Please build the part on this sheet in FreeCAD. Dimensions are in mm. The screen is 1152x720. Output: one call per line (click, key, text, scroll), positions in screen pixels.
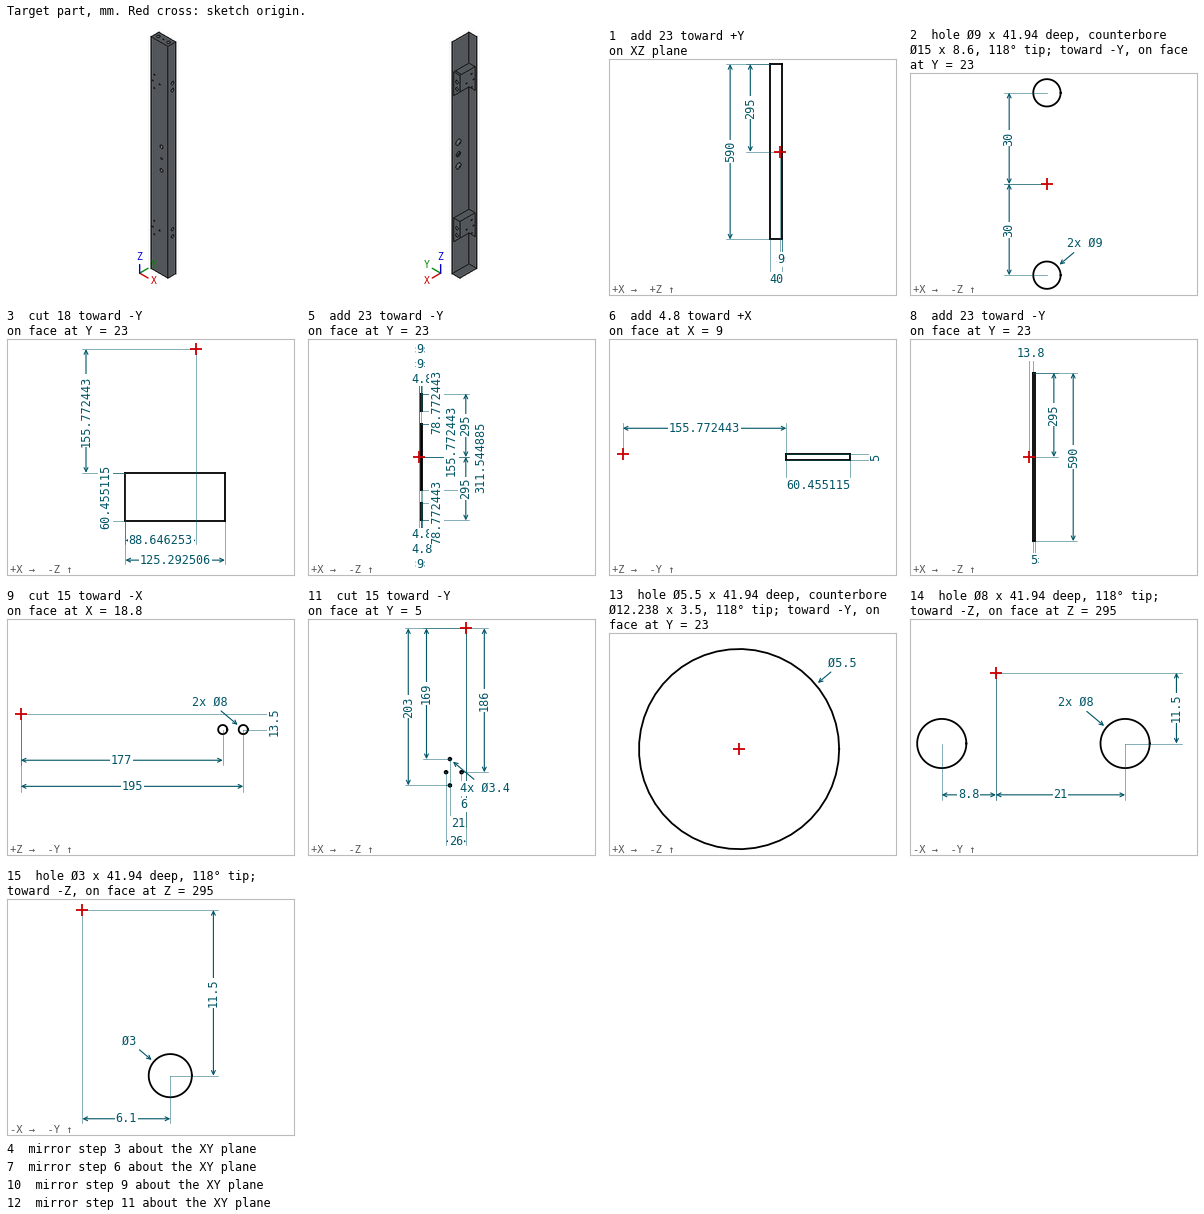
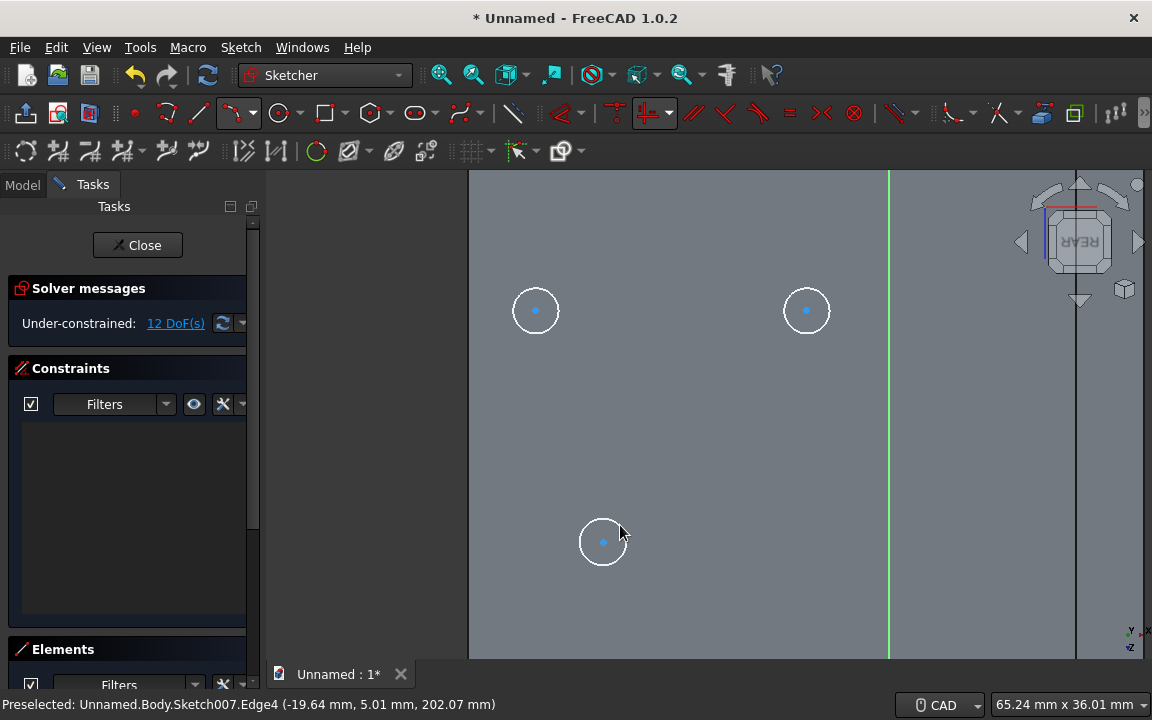
scroll(603, 542, down, 3)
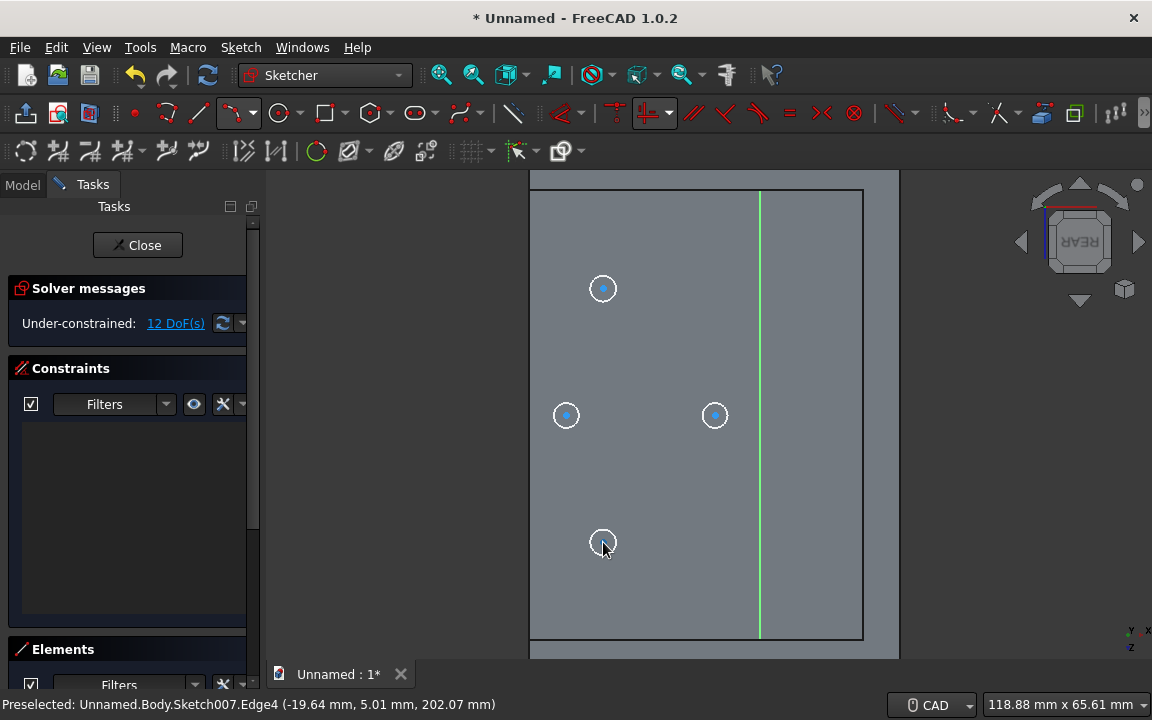
click(612, 280)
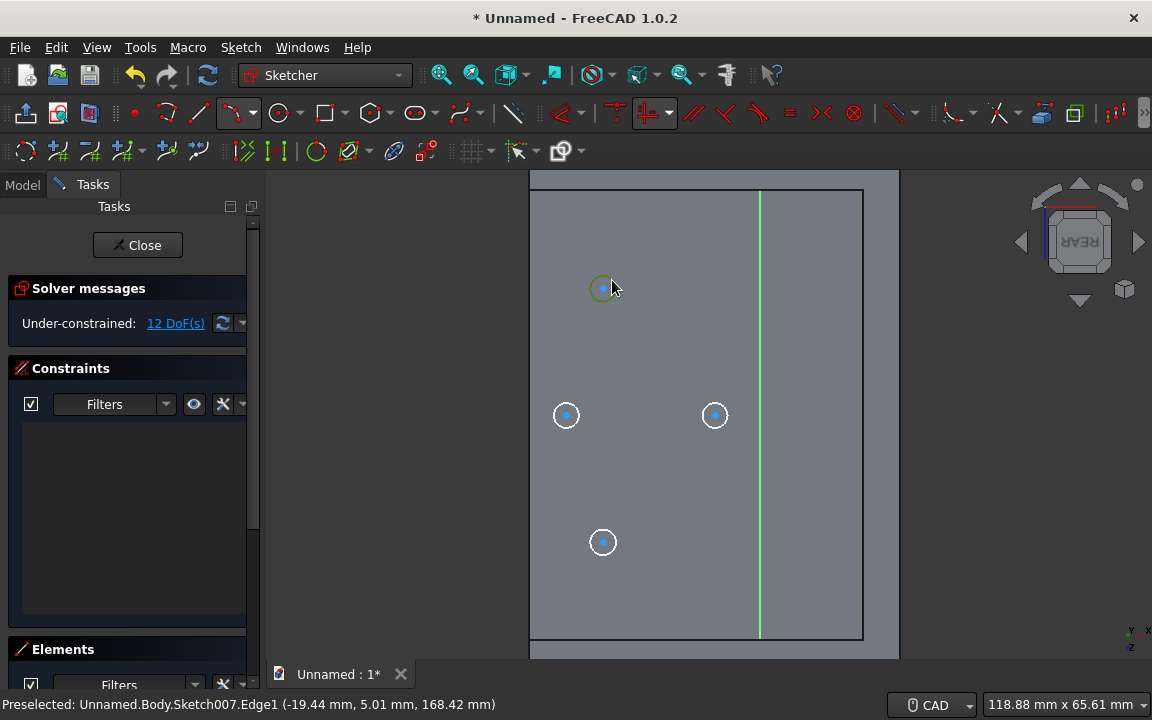
click(724, 407)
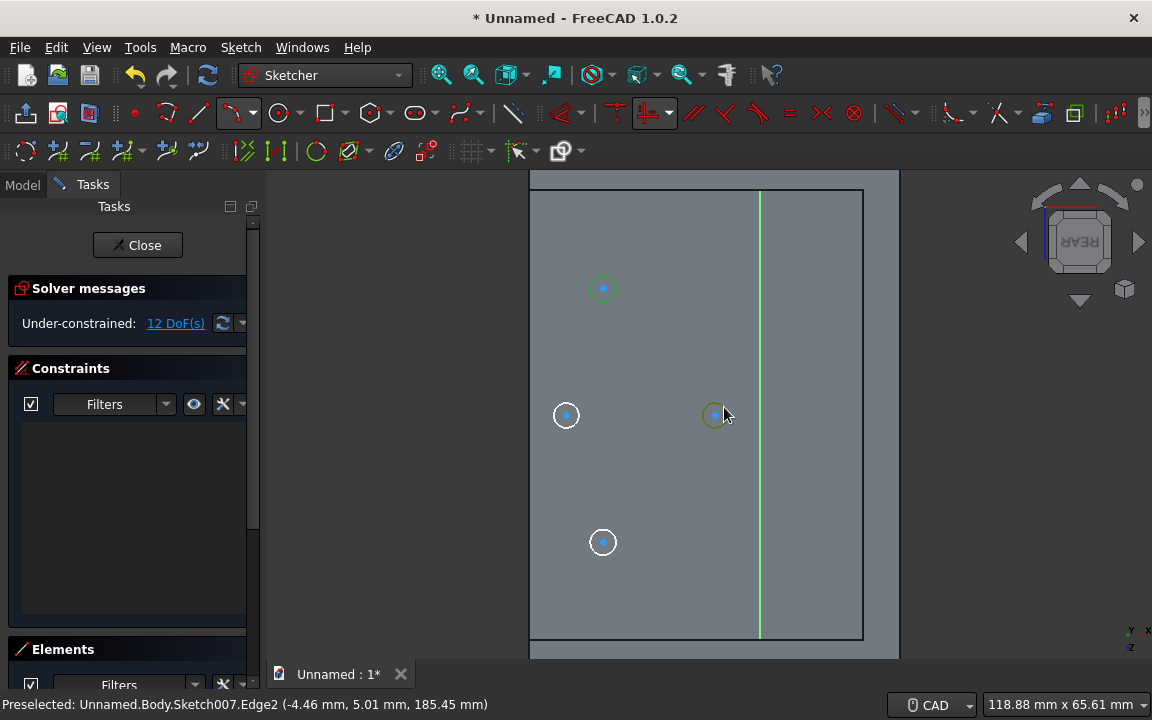
click(575, 407)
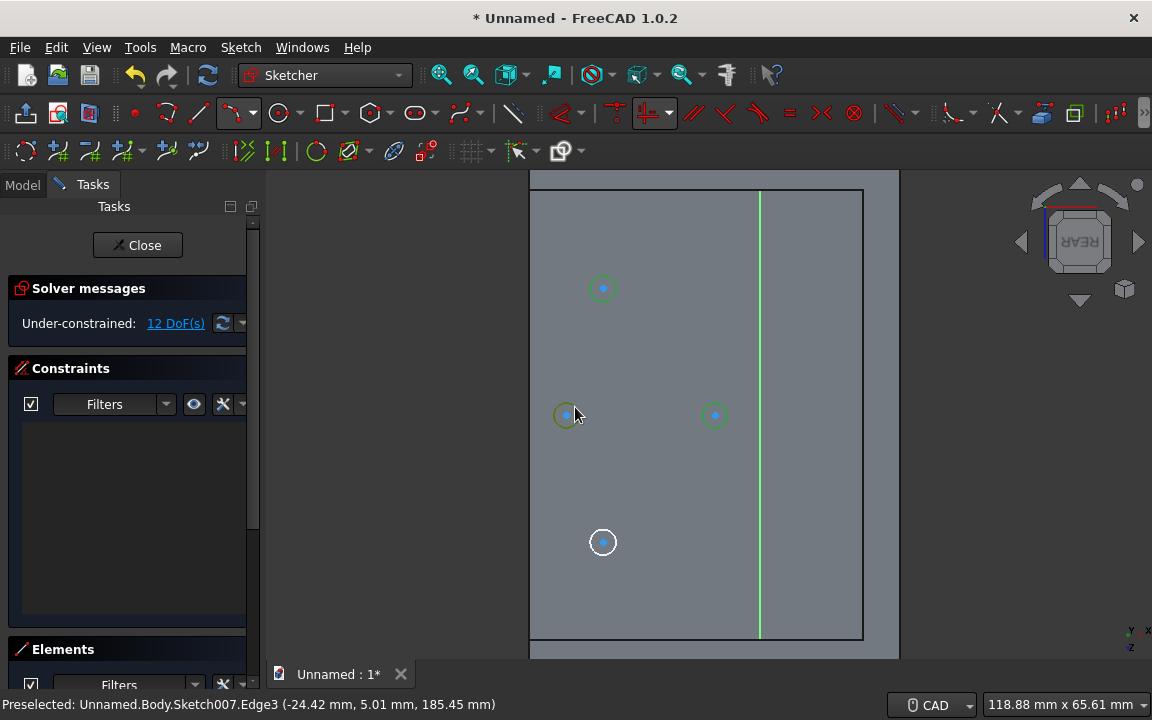
click(612, 533)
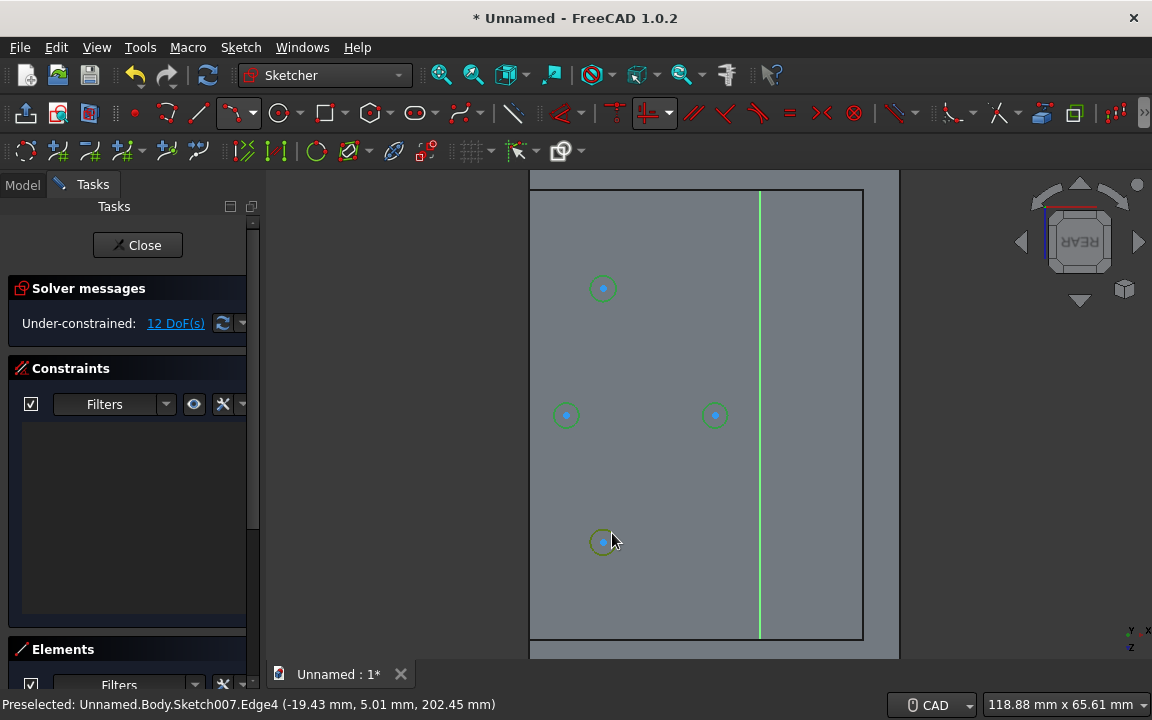
click(790, 114)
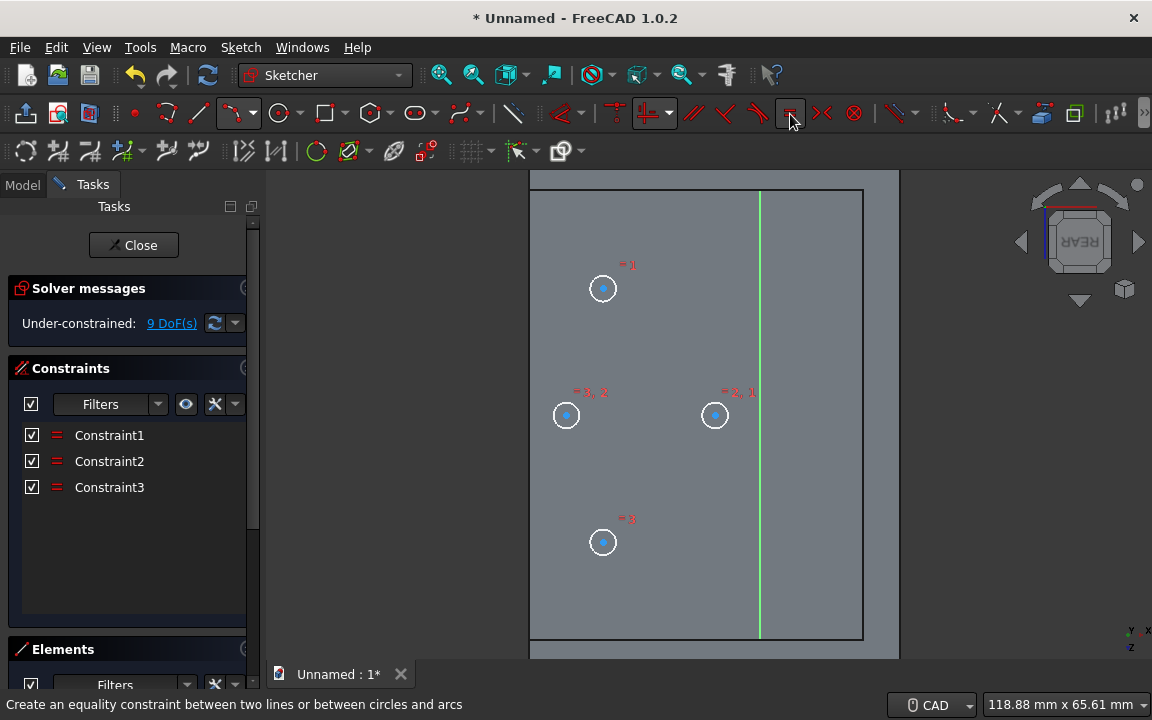
click(715, 415)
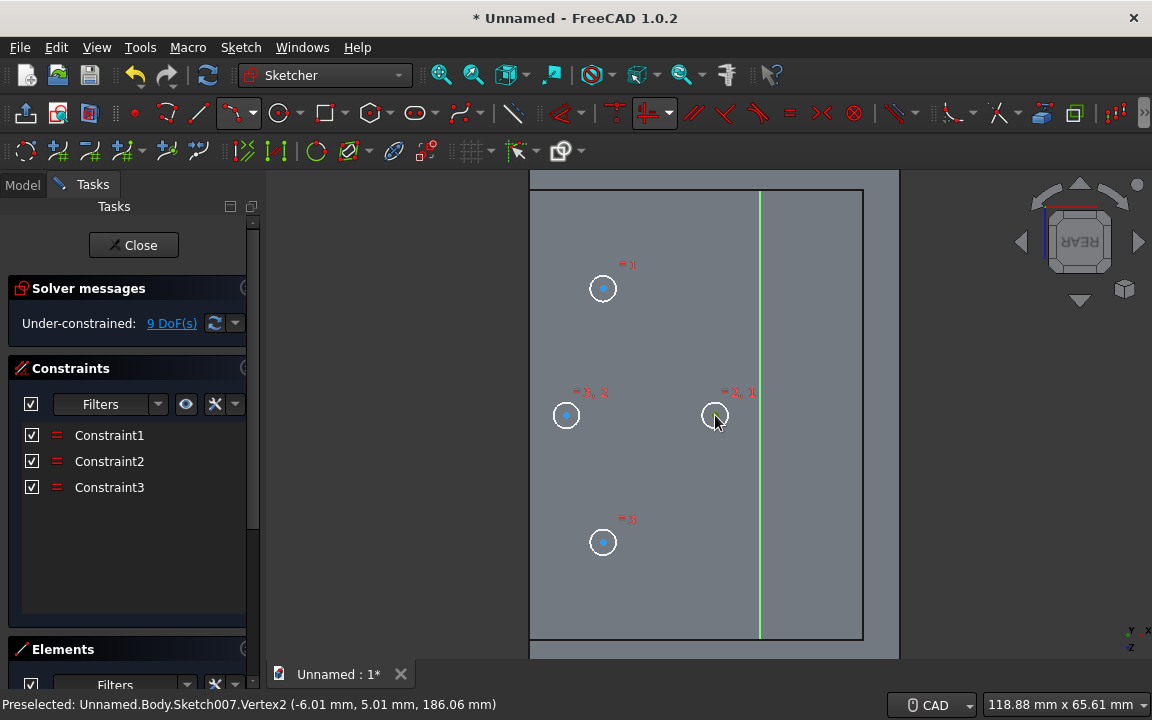
click(566, 415)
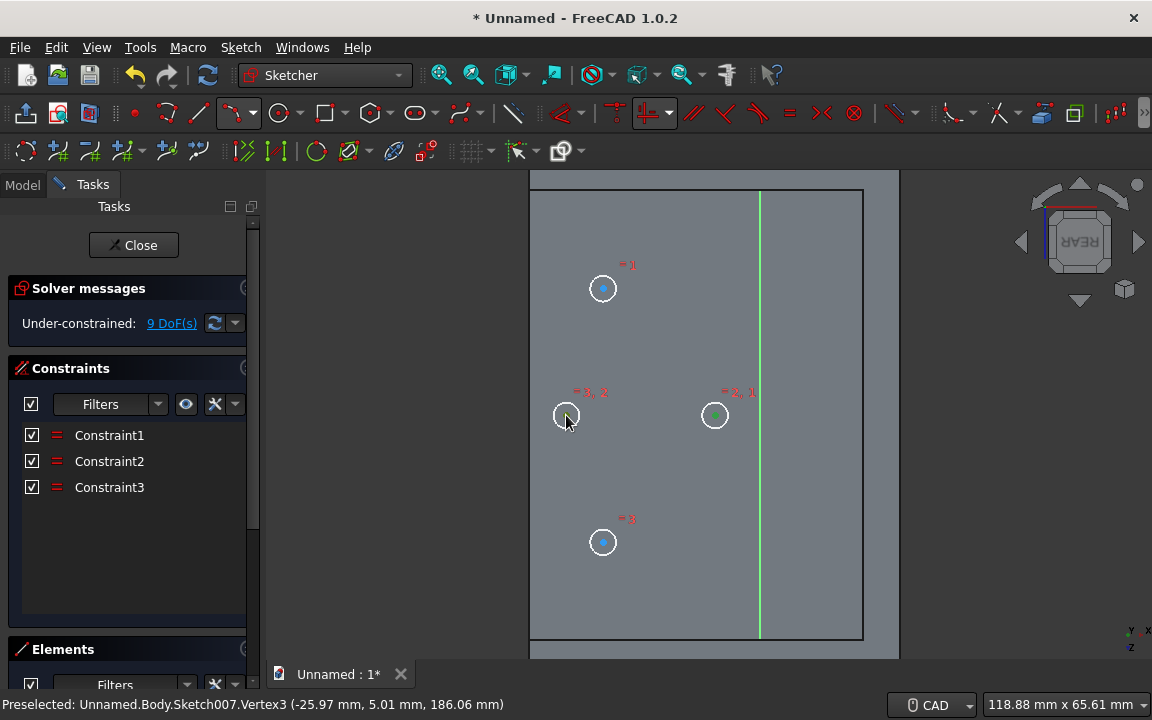
key(h)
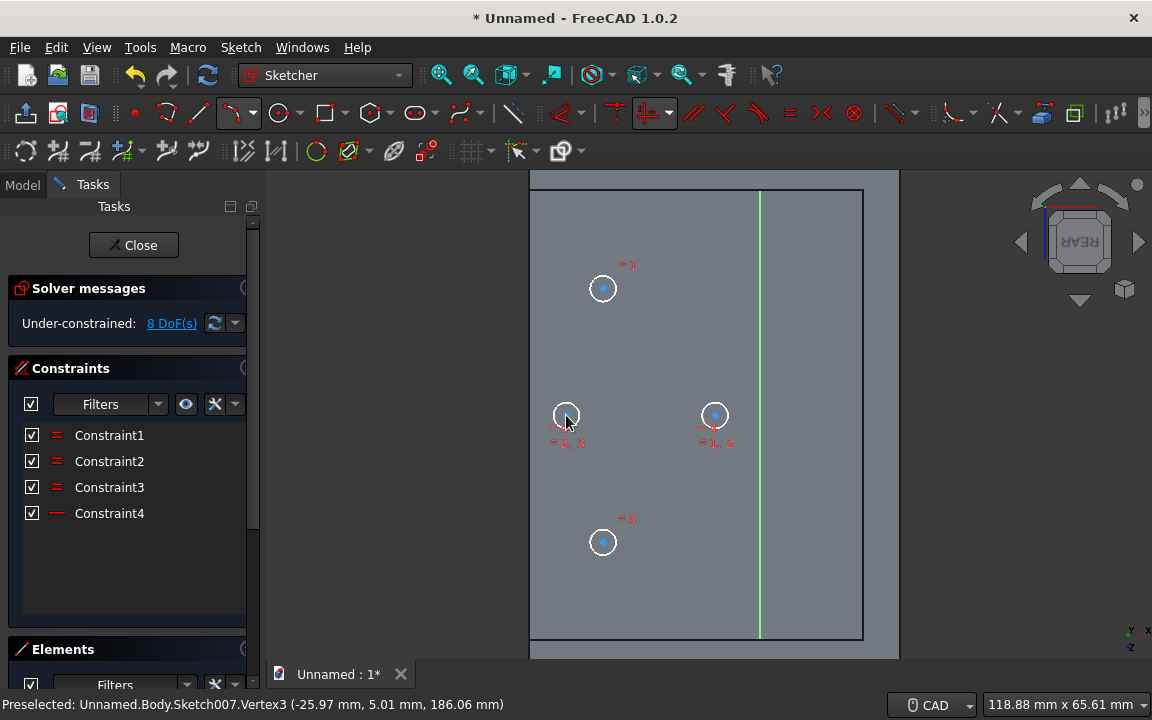
click(603, 289)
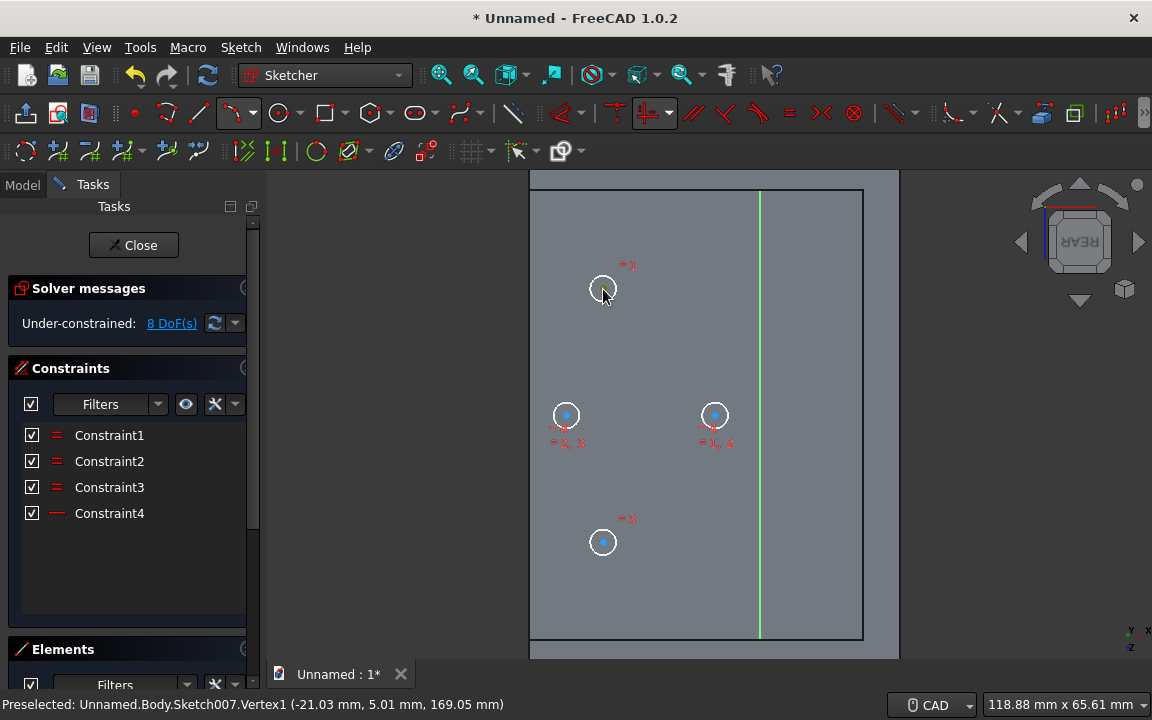
click(603, 542)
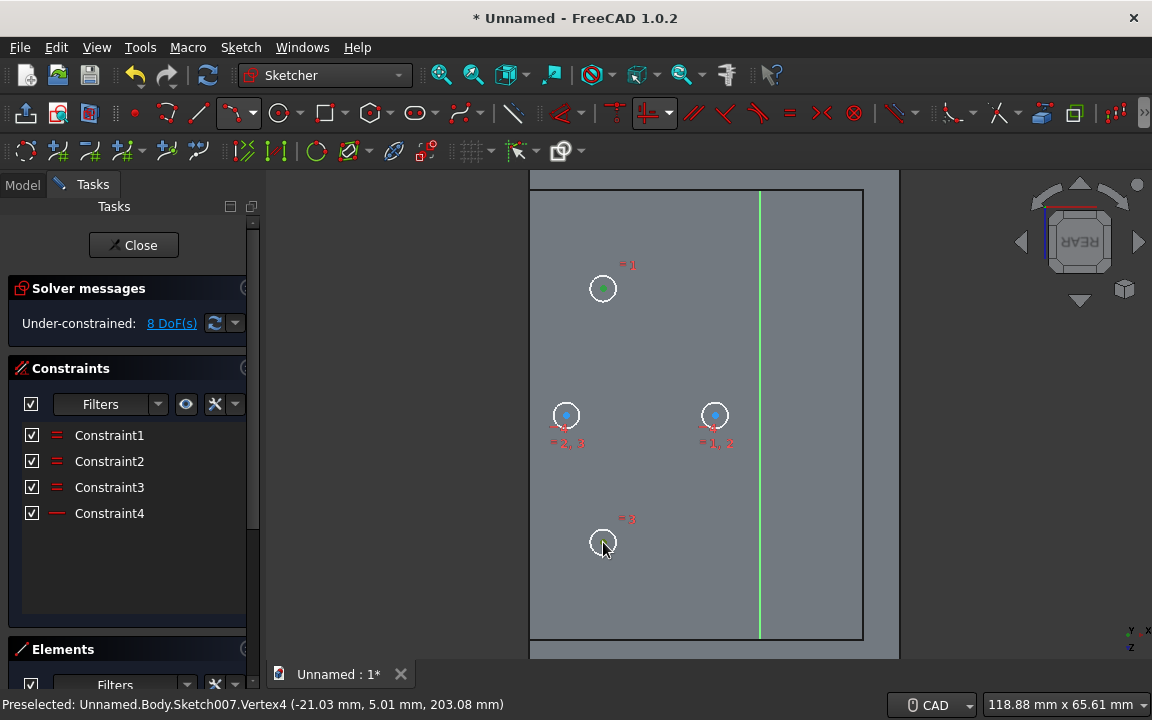
click(672, 114)